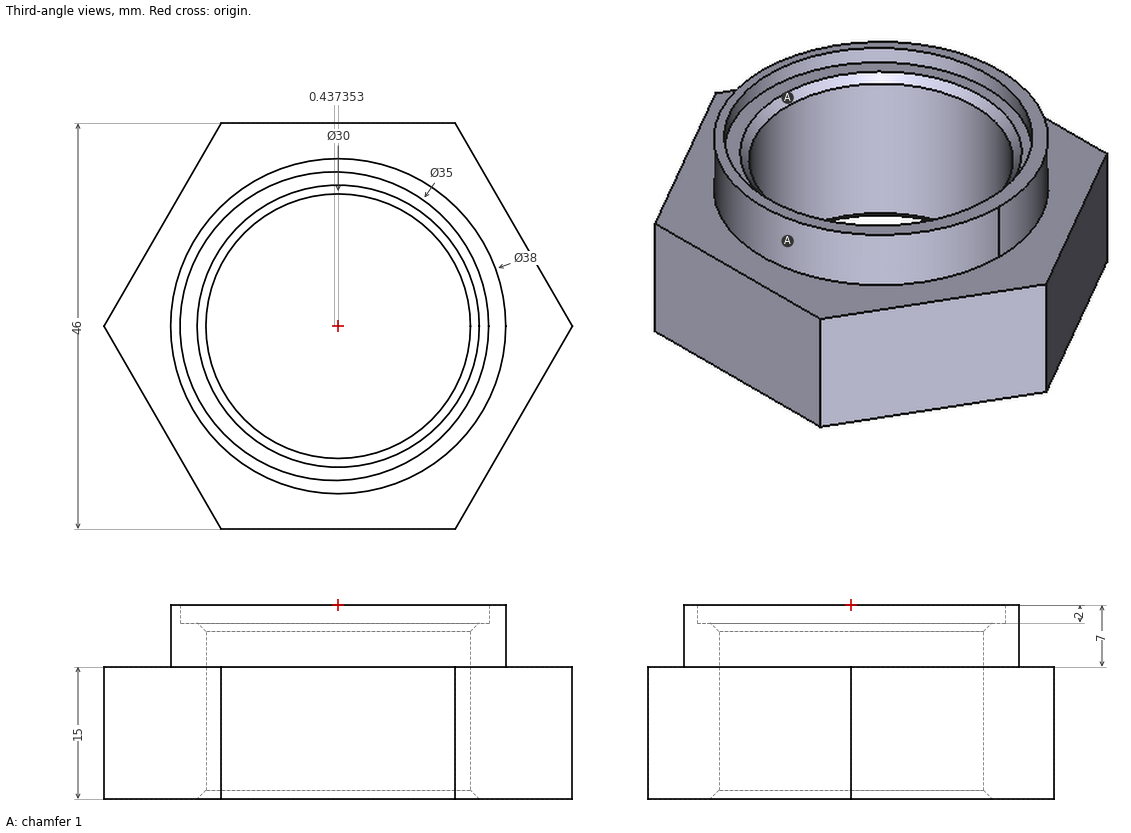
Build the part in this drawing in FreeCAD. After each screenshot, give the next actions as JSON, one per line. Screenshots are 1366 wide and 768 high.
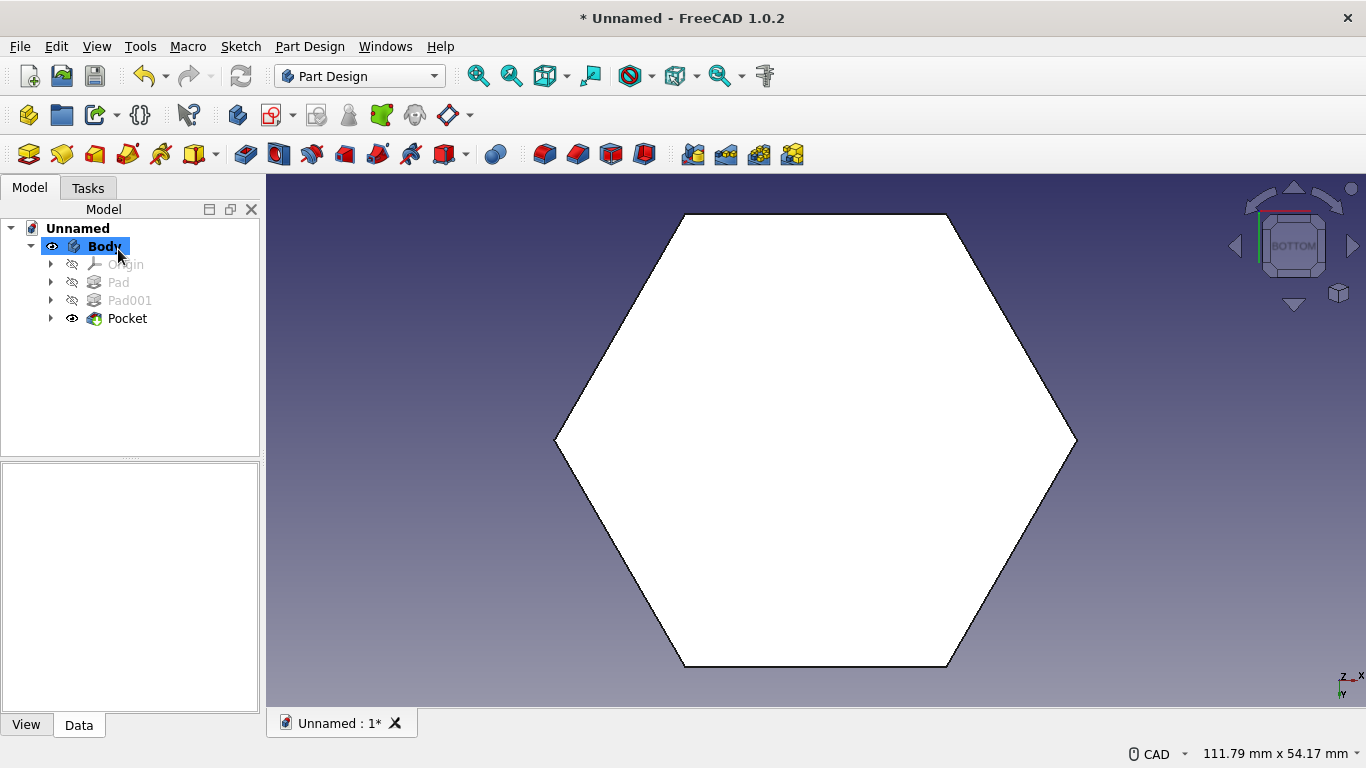
{"action": "key", "text": "0"}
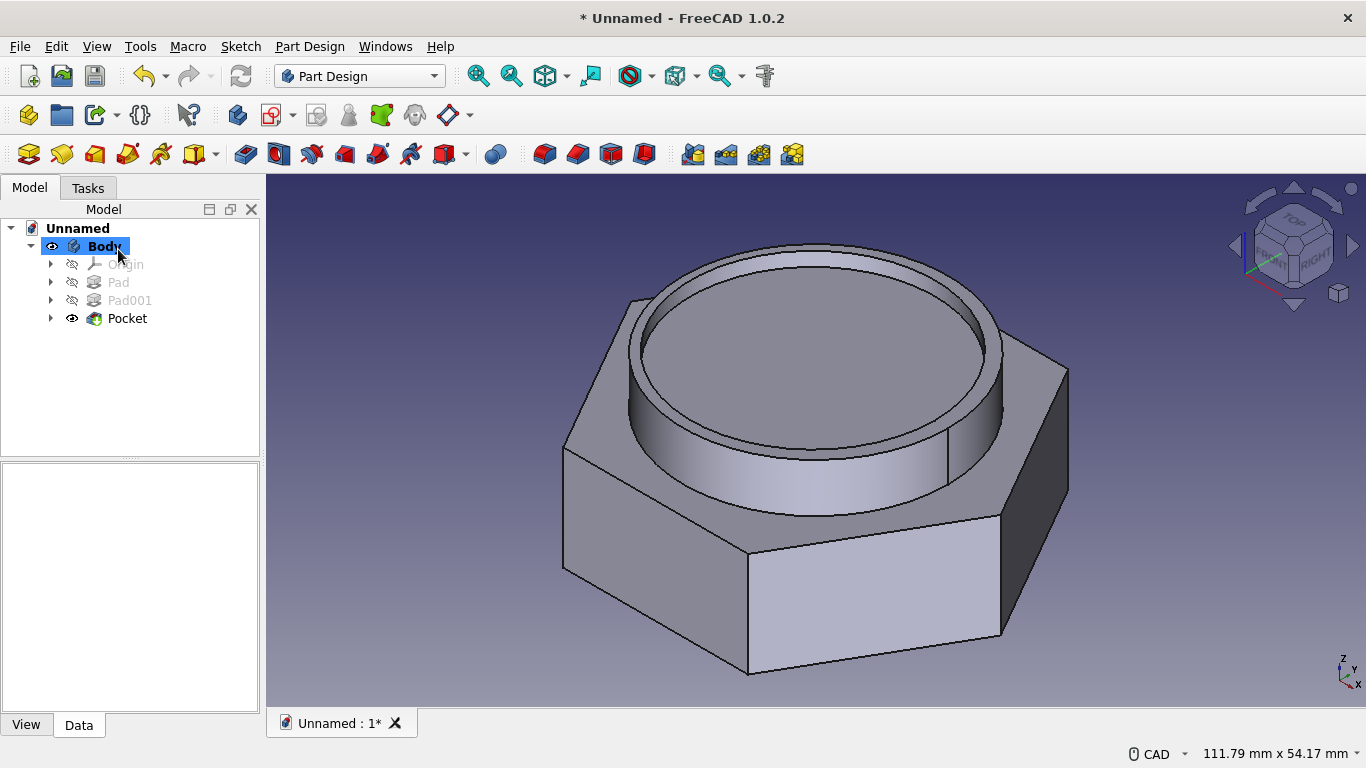
{"action": "left_click", "coordinate": [479, 76]}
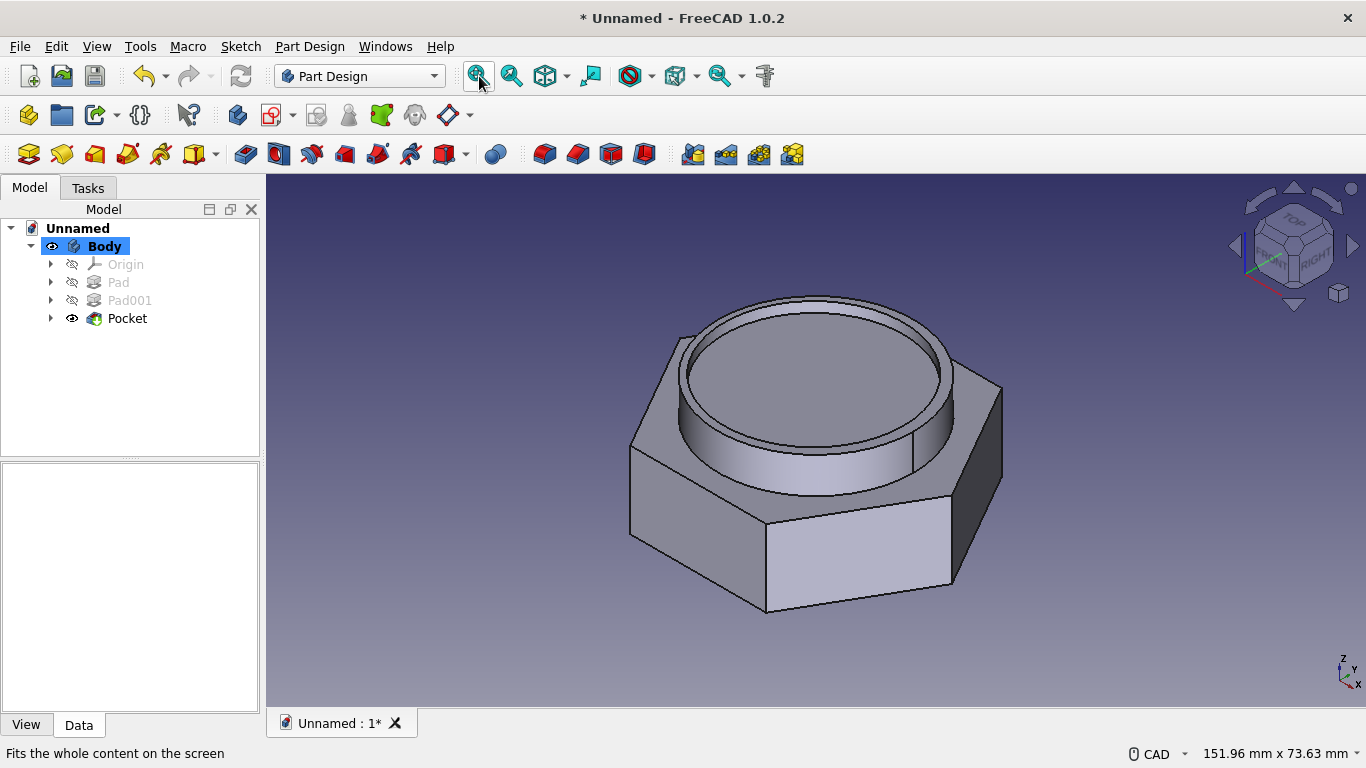
{"action": "left_click", "coordinate": [814, 385]}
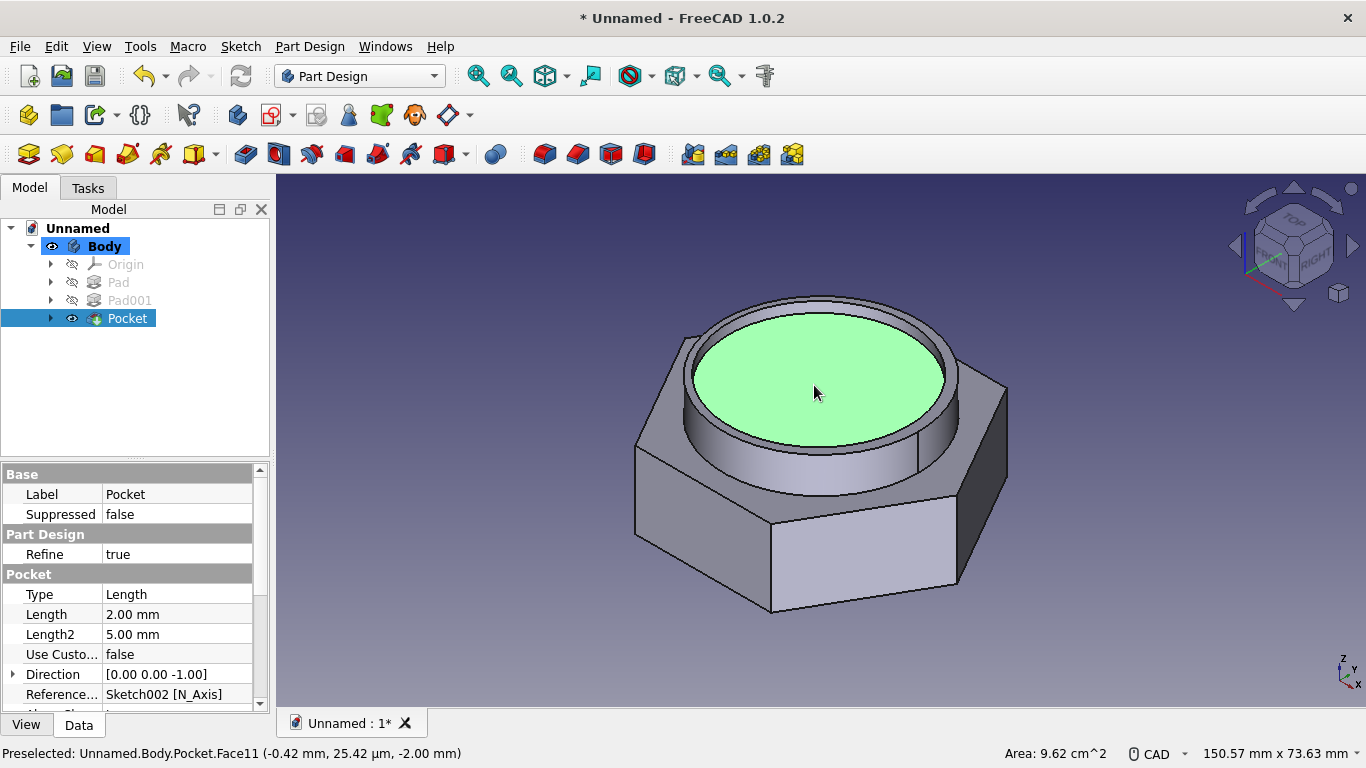
{"action": "left_click", "coordinate": [270, 116]}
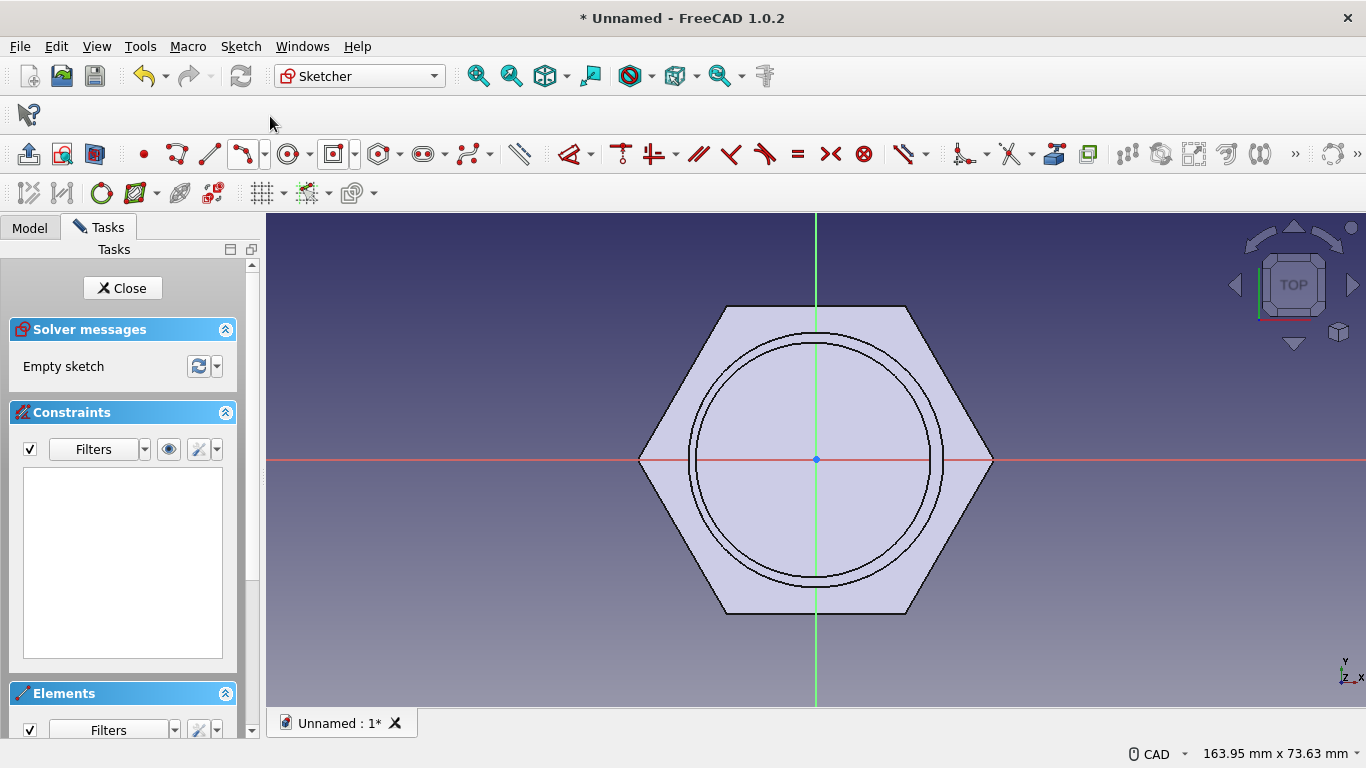
{"action": "scroll", "coordinate": [955, 460], "scroll_direction": "up", "scroll_amount": 2}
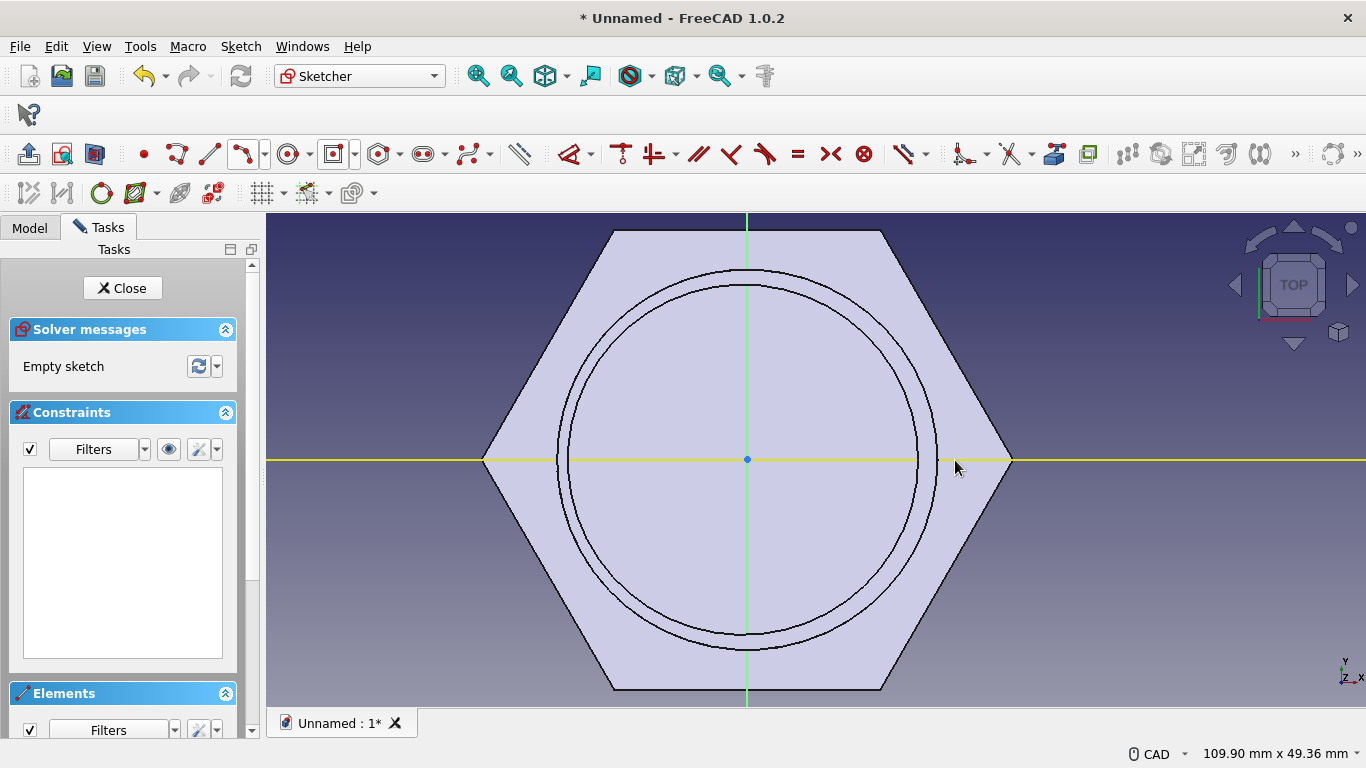
{"action": "left_click", "coordinate": [288, 154]}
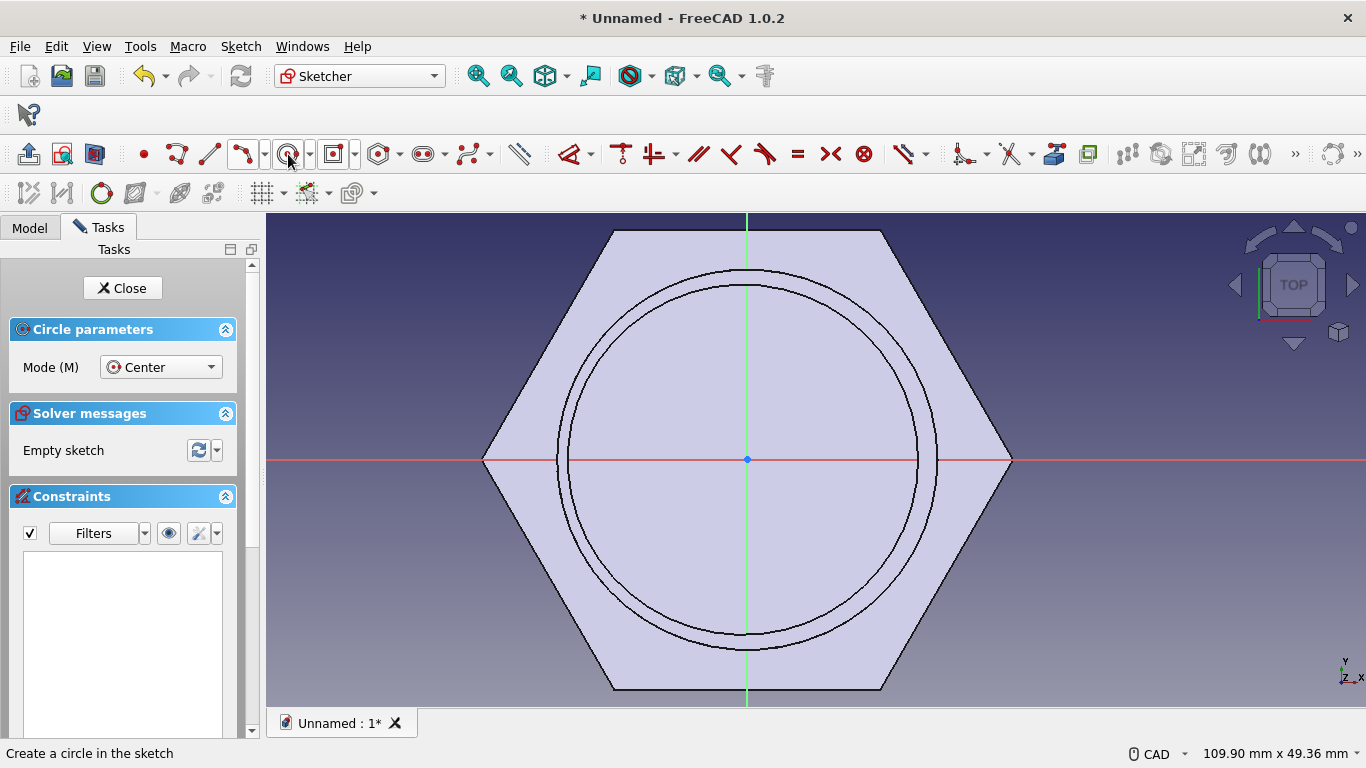
{"action": "left_click", "coordinate": [747, 460]}
{"action": "mouse_move", "coordinate": [853, 354]}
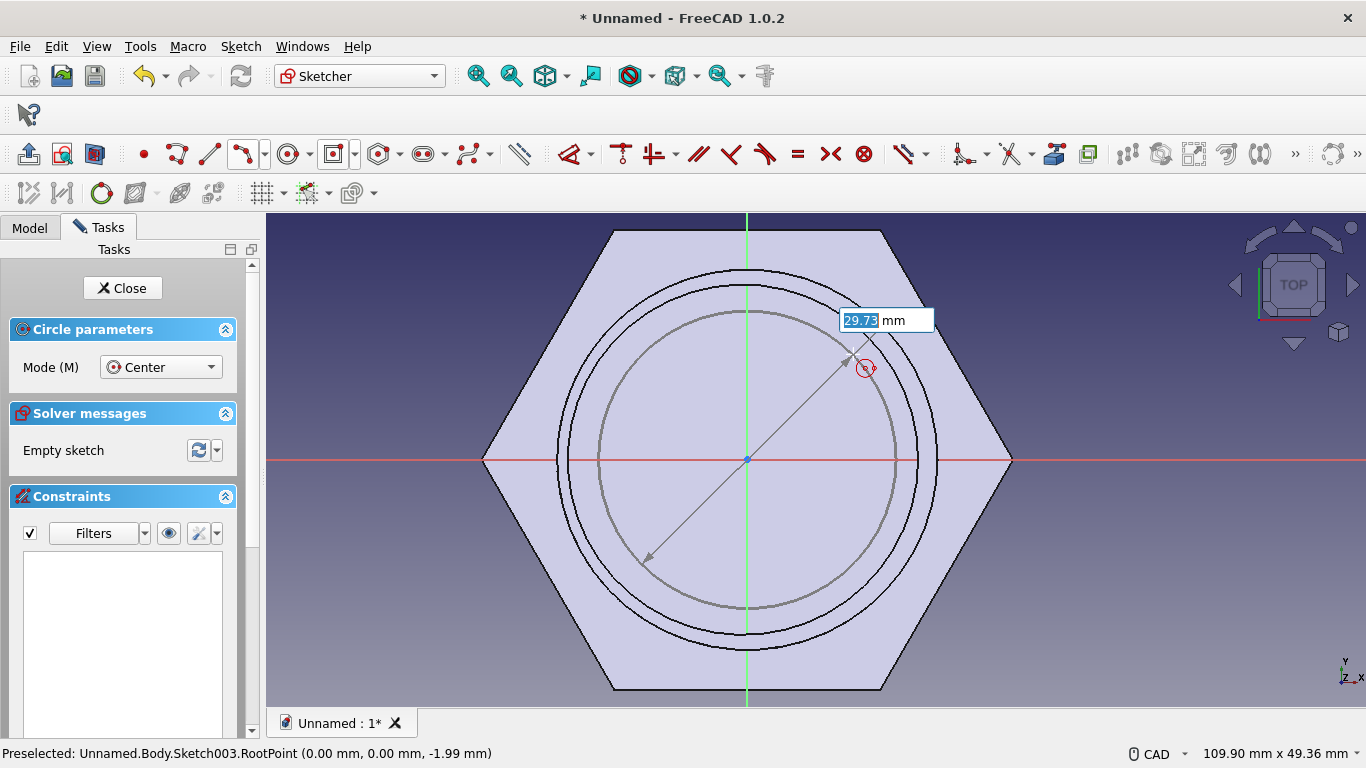
{"action": "type", "text": "30"}
{"action": "key", "text": "Return"}
{"action": "key", "text": "Escape"}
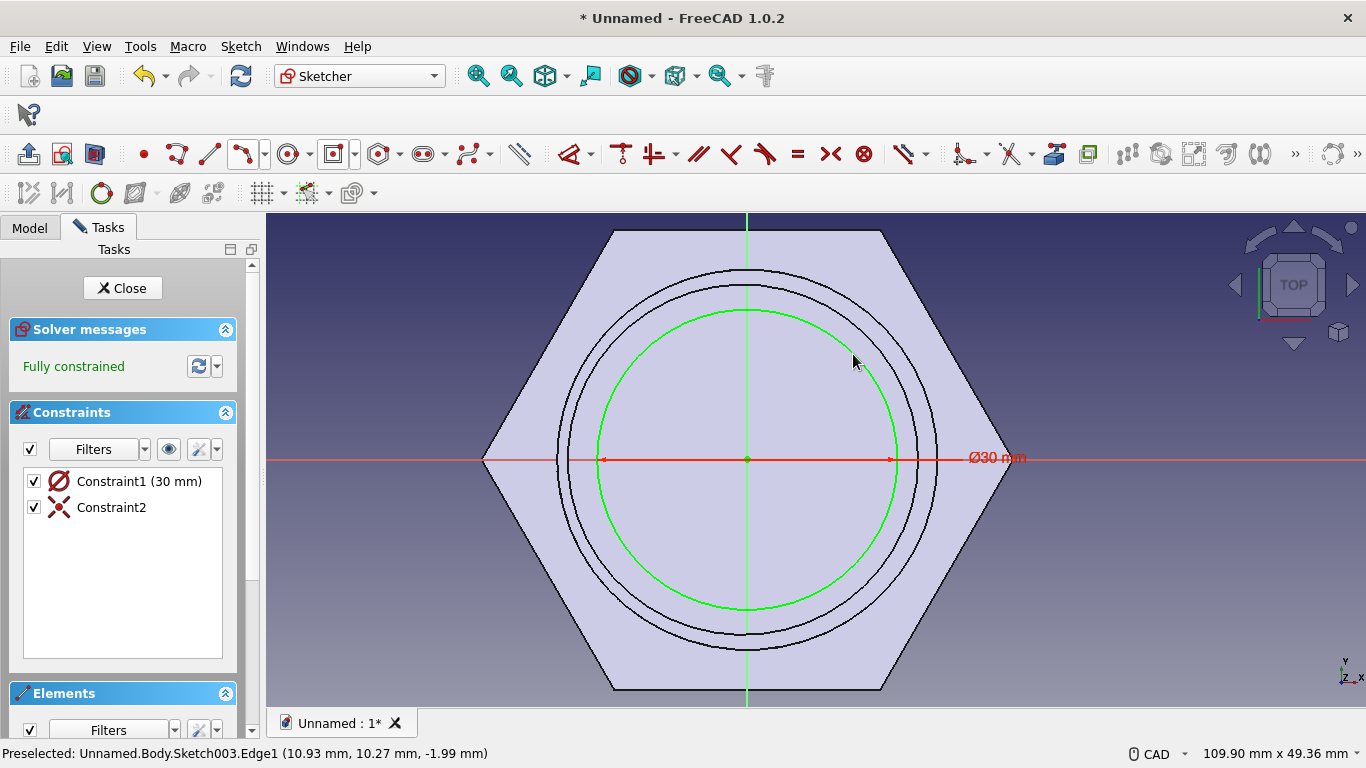
{"action": "left_click", "coordinate": [123, 288]}